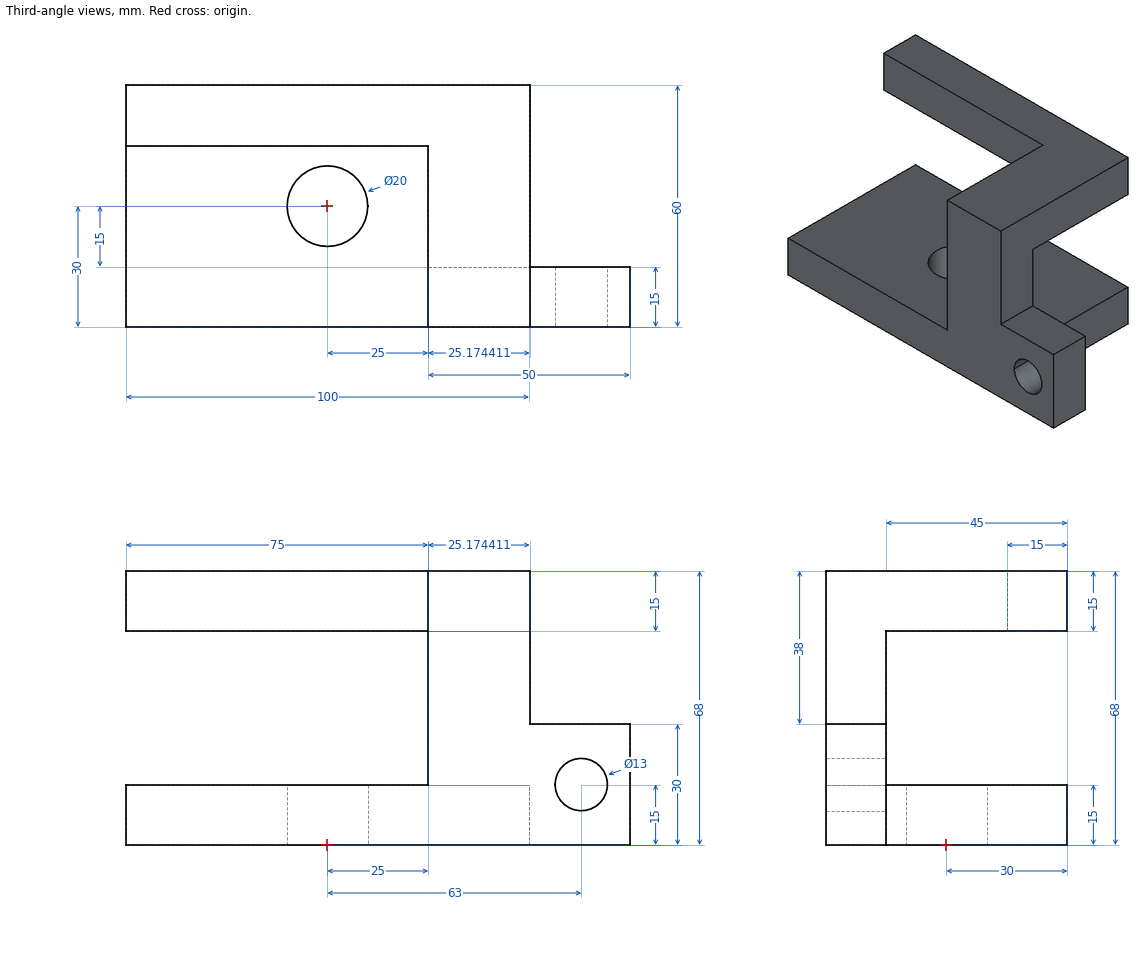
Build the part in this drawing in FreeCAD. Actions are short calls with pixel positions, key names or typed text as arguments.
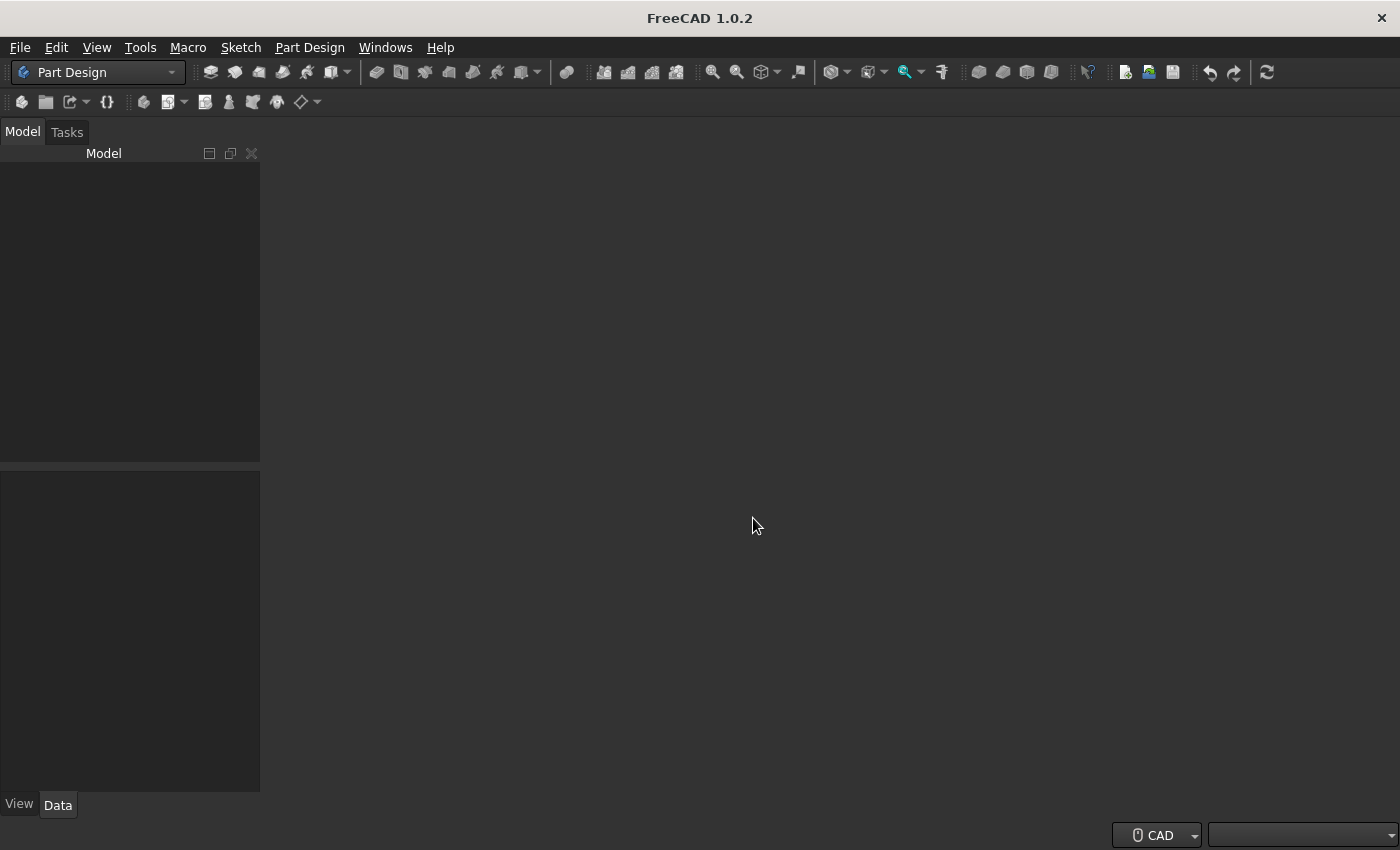
click(1126, 72)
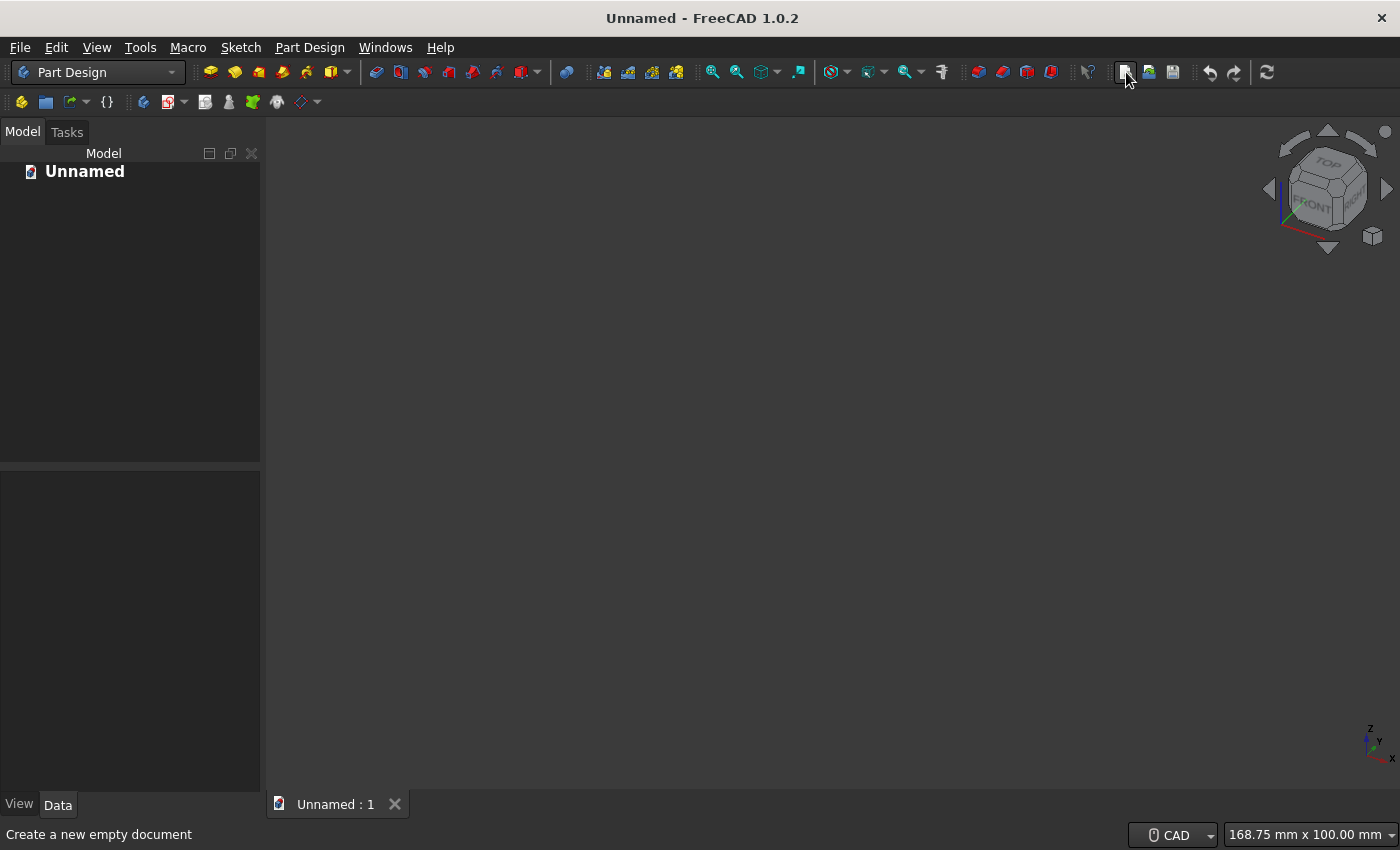
click(168, 102)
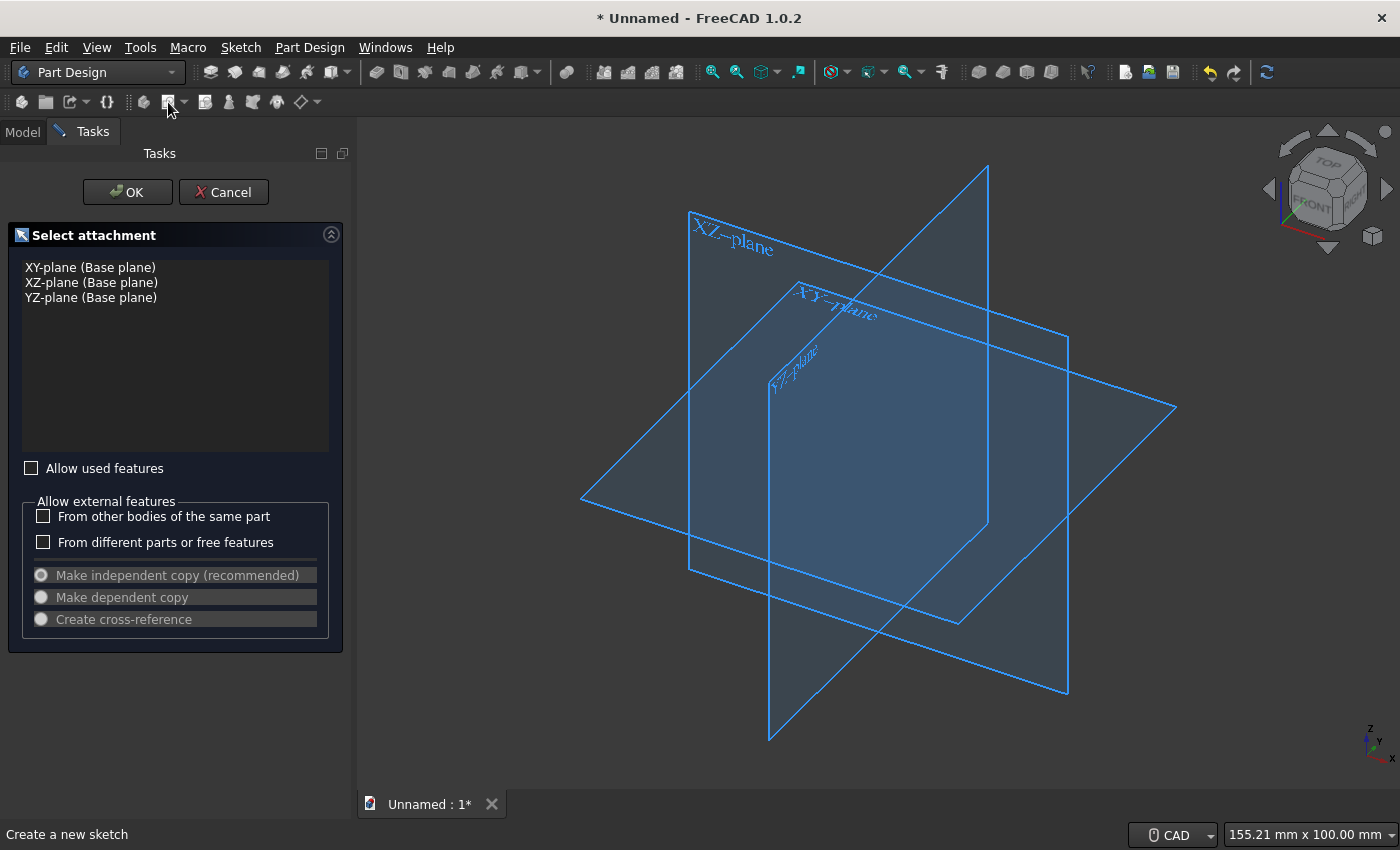
click(82, 268)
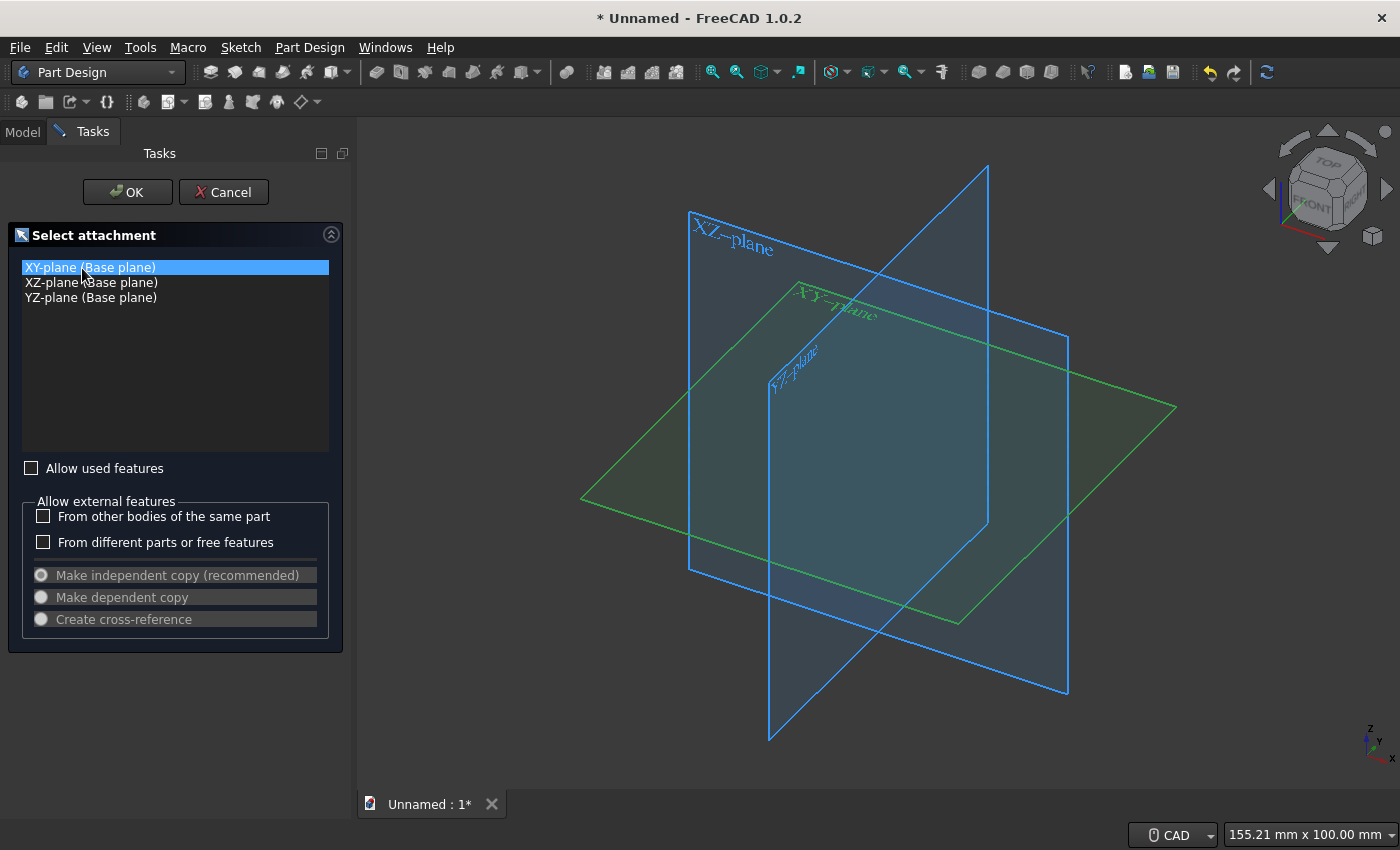
click(128, 192)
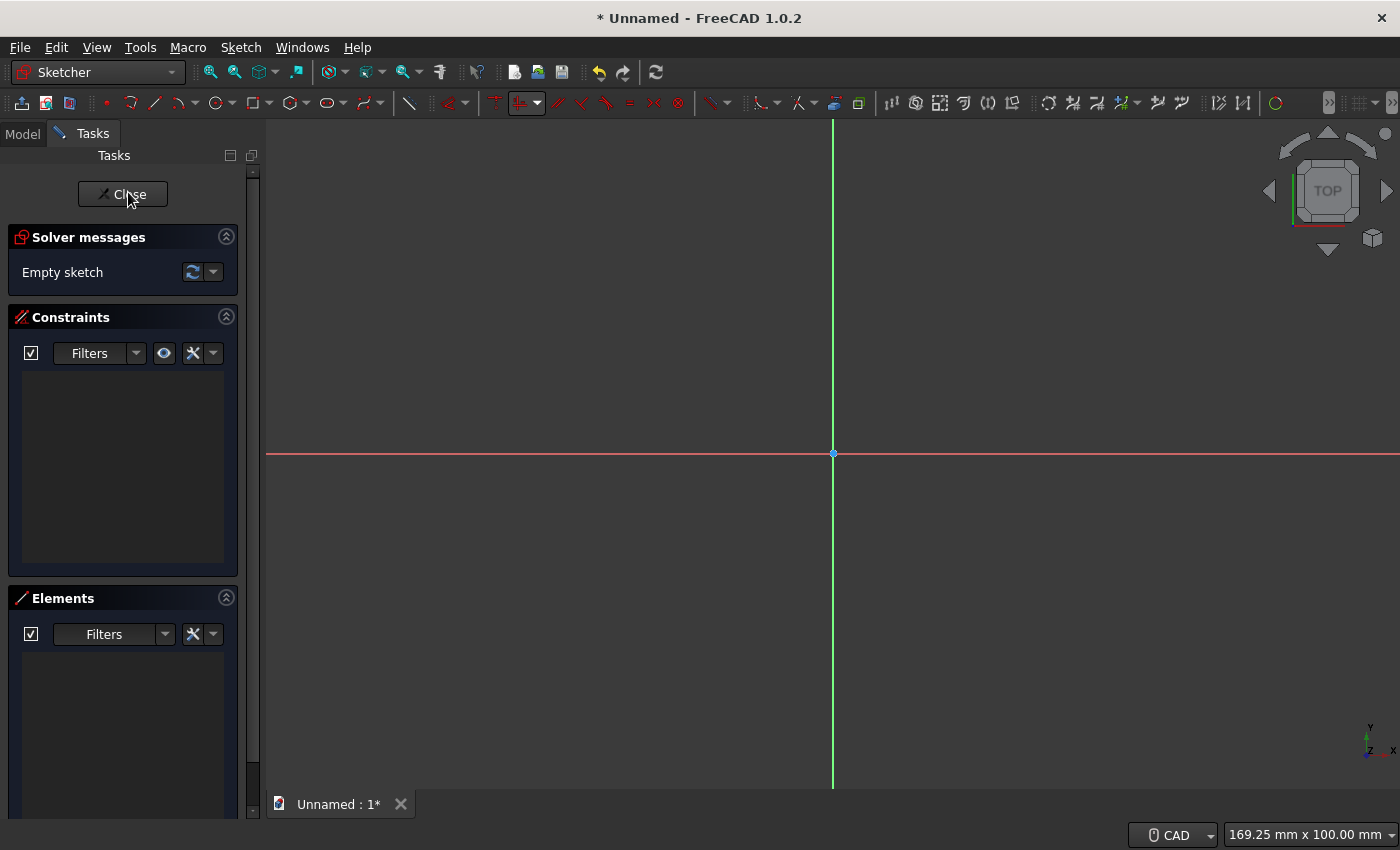
click(272, 104)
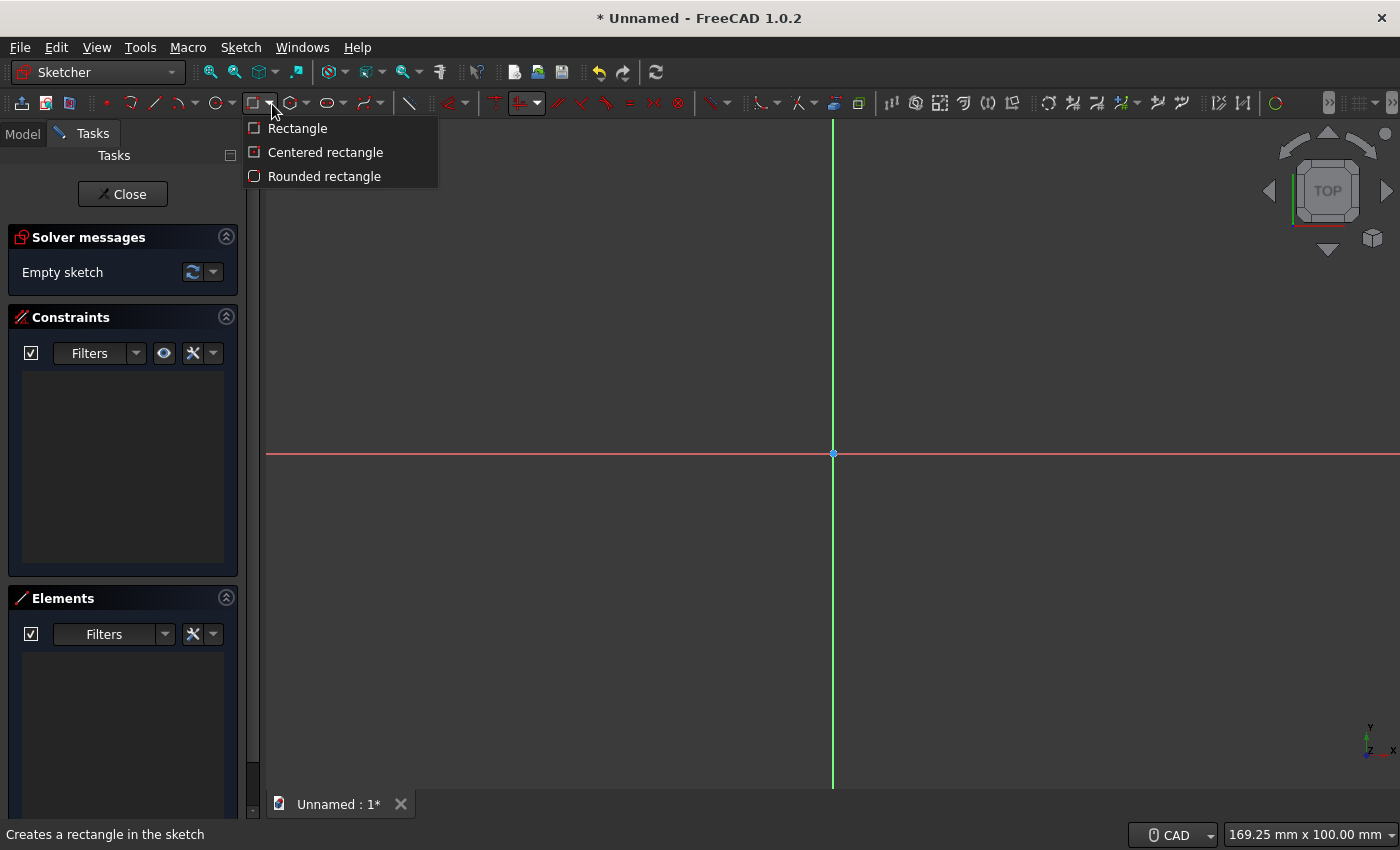
click(340, 152)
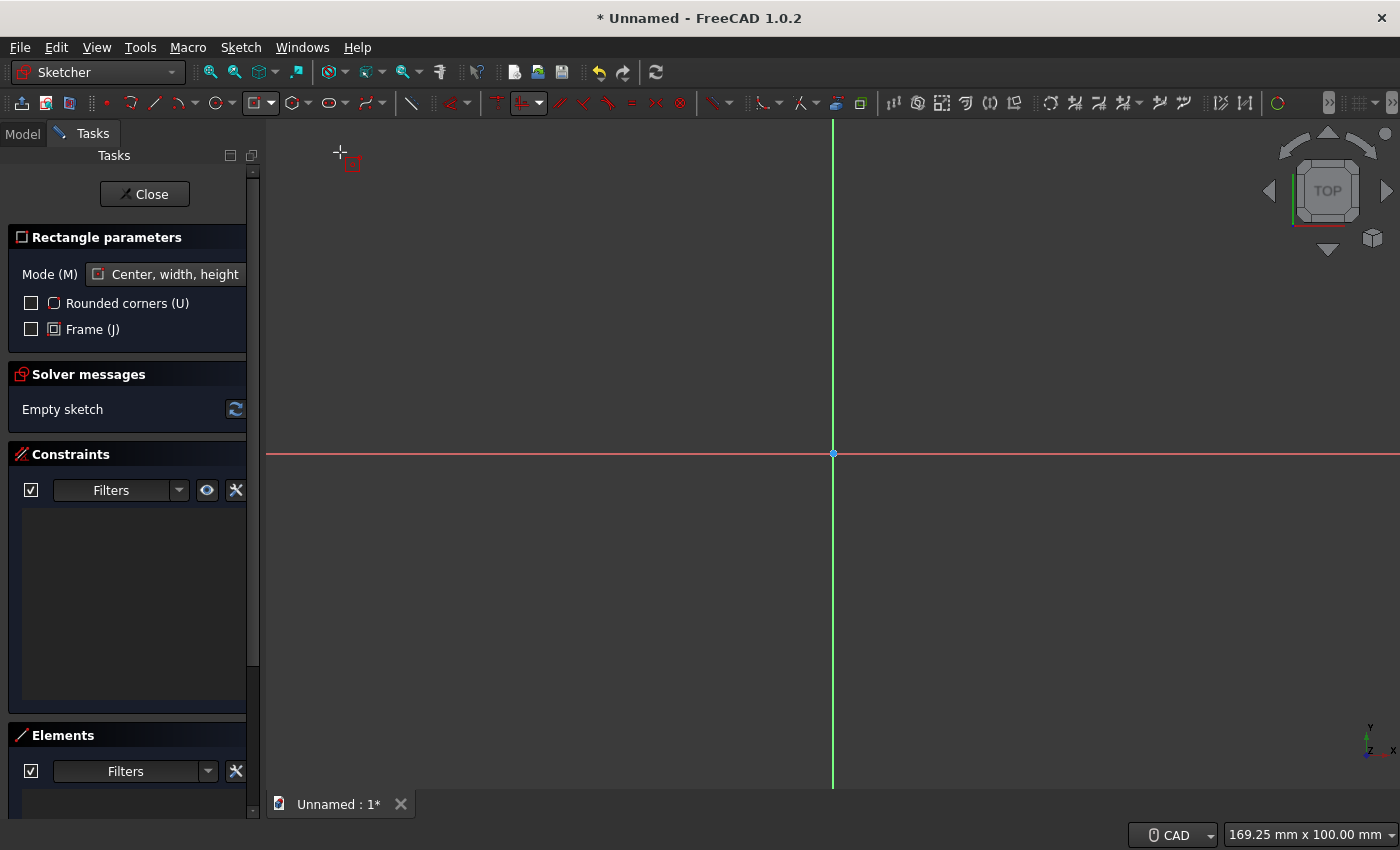
click(833, 454)
move(1168, 253)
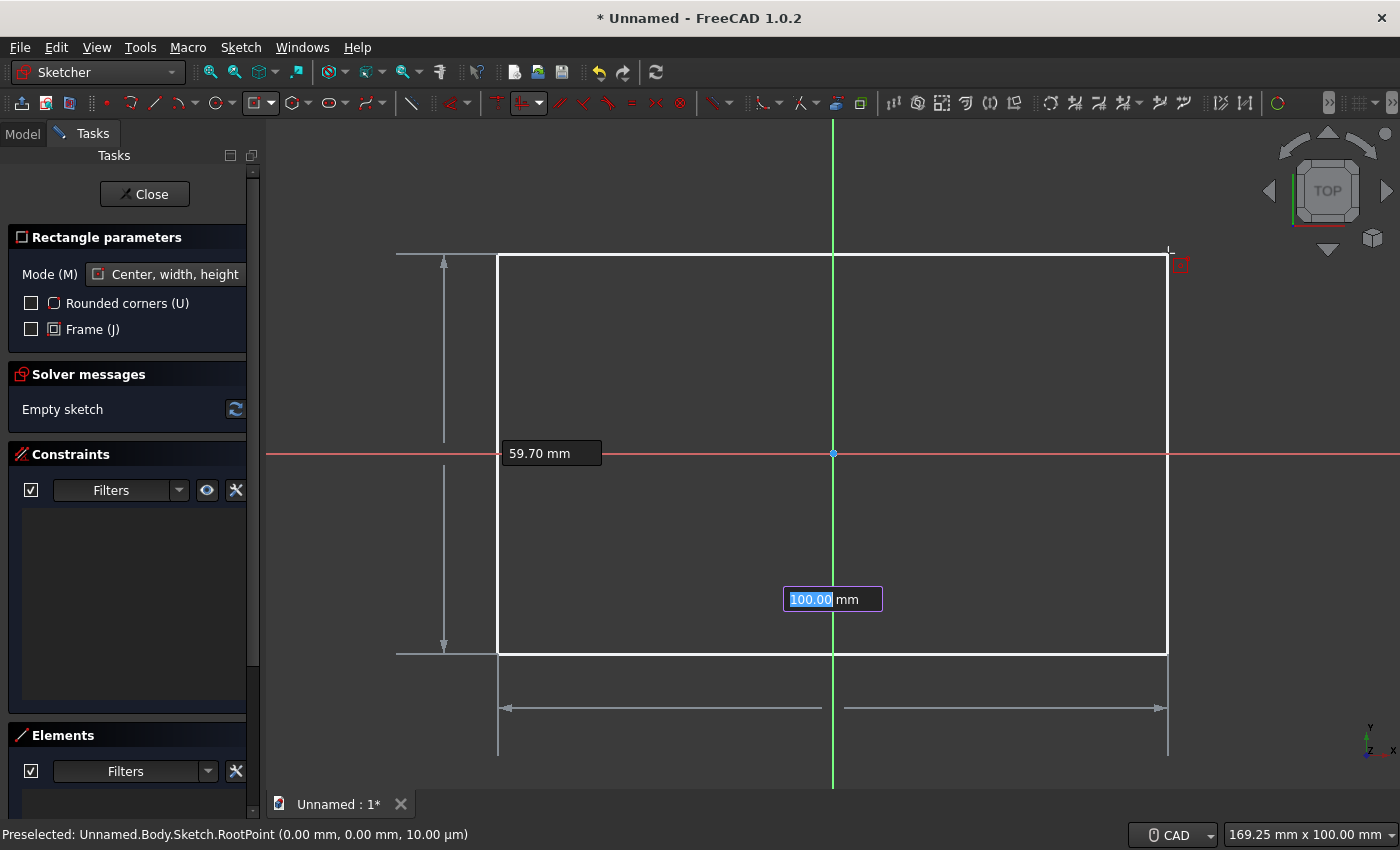
text(100)
key(Tab)
text(60)
key(Return)
key(Escape)